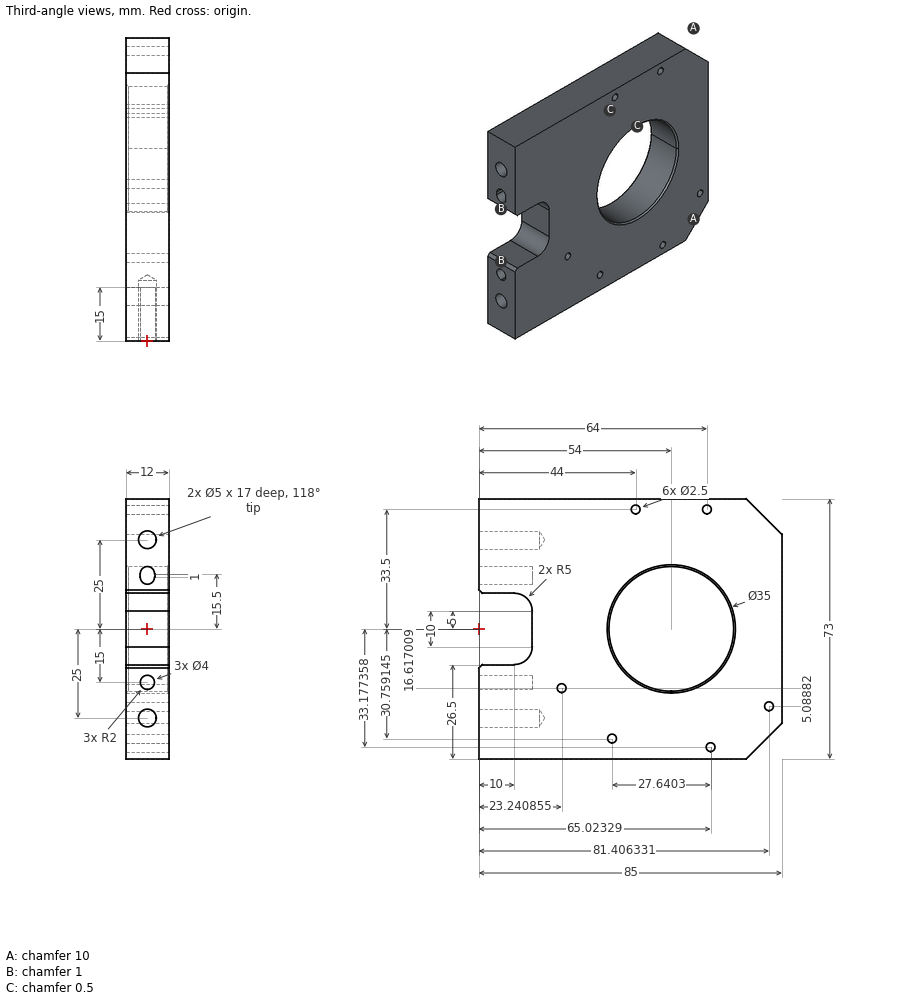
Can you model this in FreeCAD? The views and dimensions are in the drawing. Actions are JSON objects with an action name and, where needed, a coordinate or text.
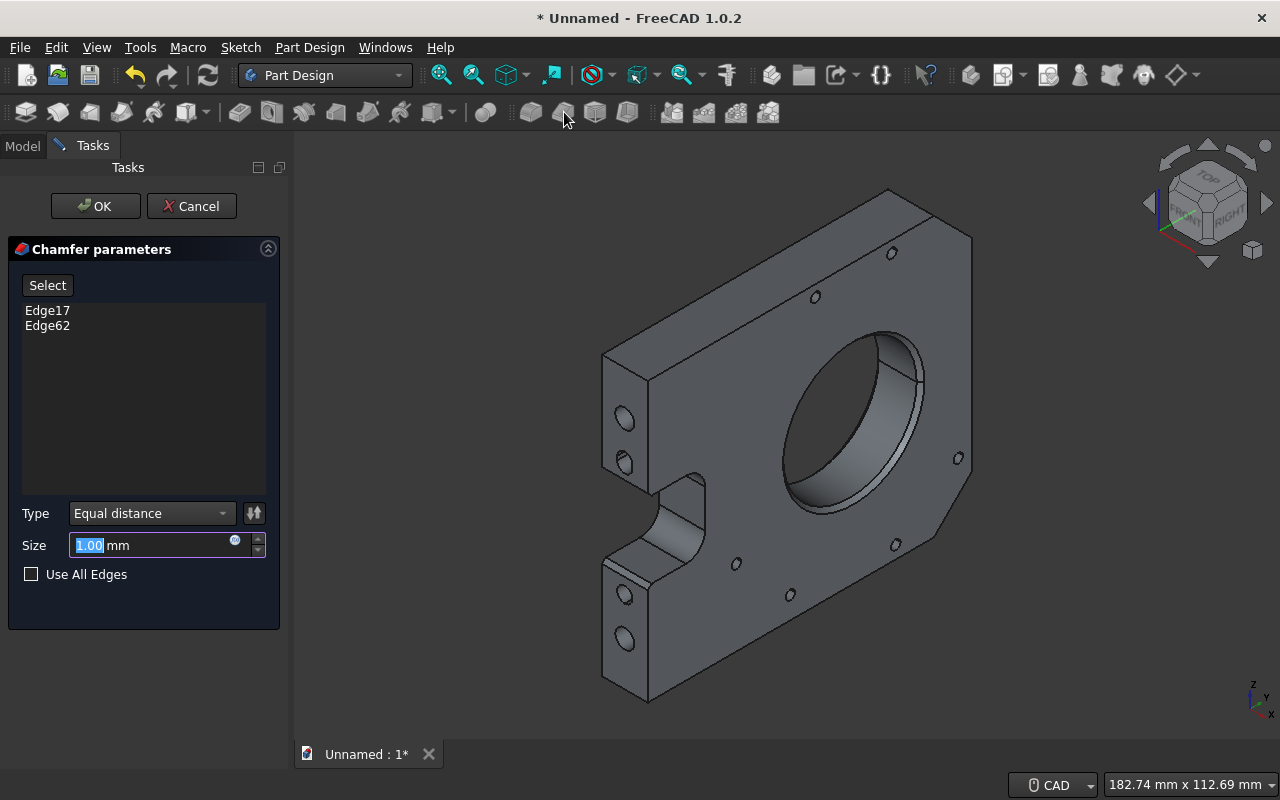
{"action": "type", "text": "0.5"}
{"action": "key", "text": "Tab"}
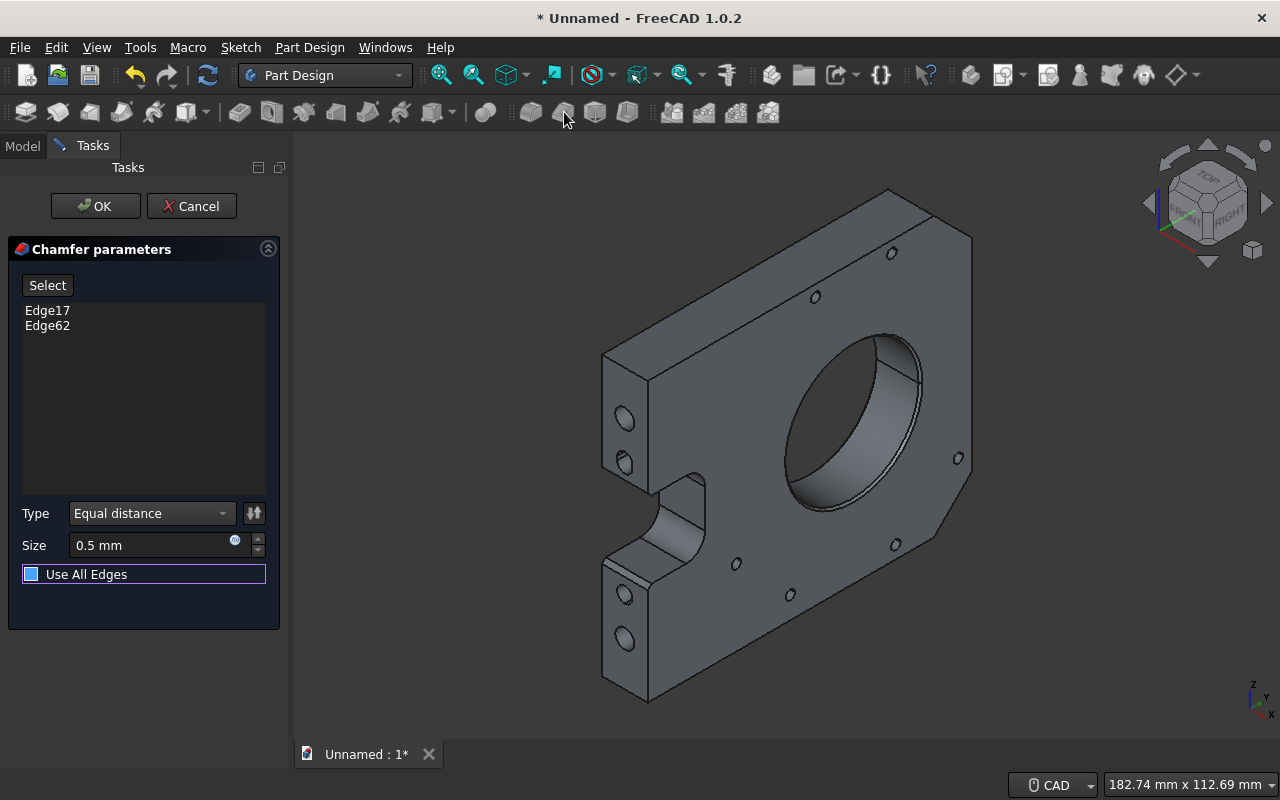
{"action": "left_click", "coordinate": [96, 206]}